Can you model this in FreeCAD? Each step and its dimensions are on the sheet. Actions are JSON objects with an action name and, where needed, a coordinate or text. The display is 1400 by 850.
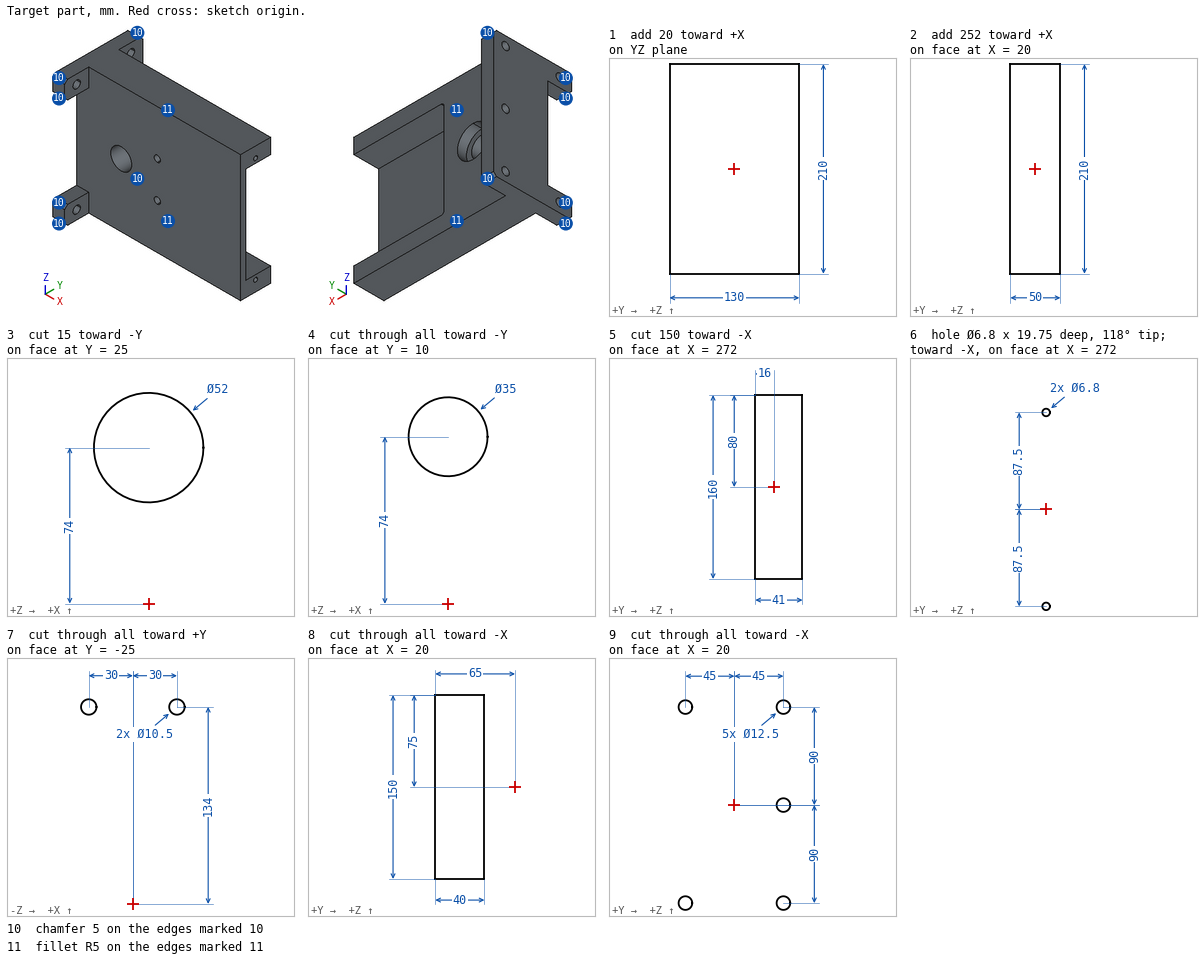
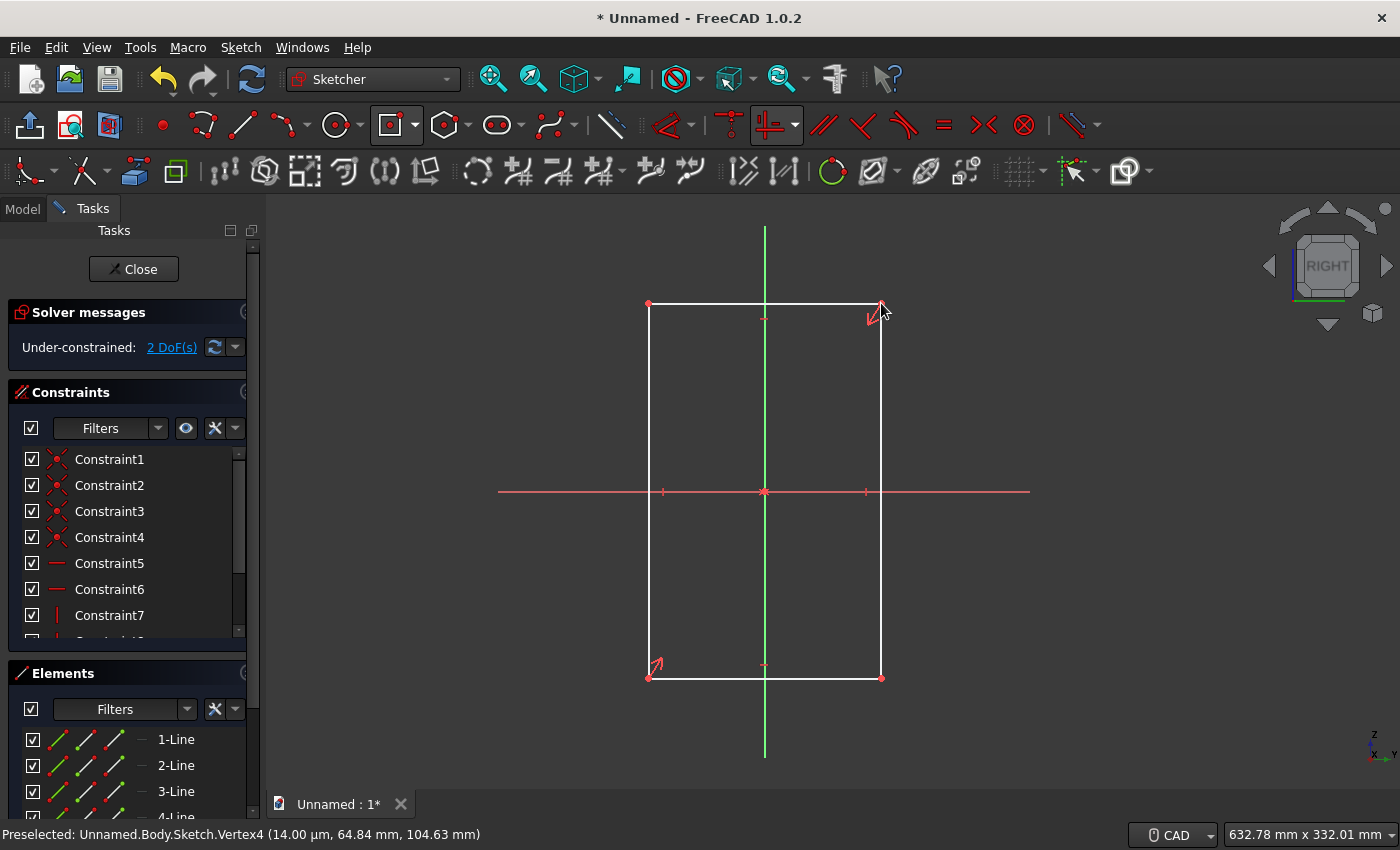
{"action": "left_click", "coordinate": [666, 126]}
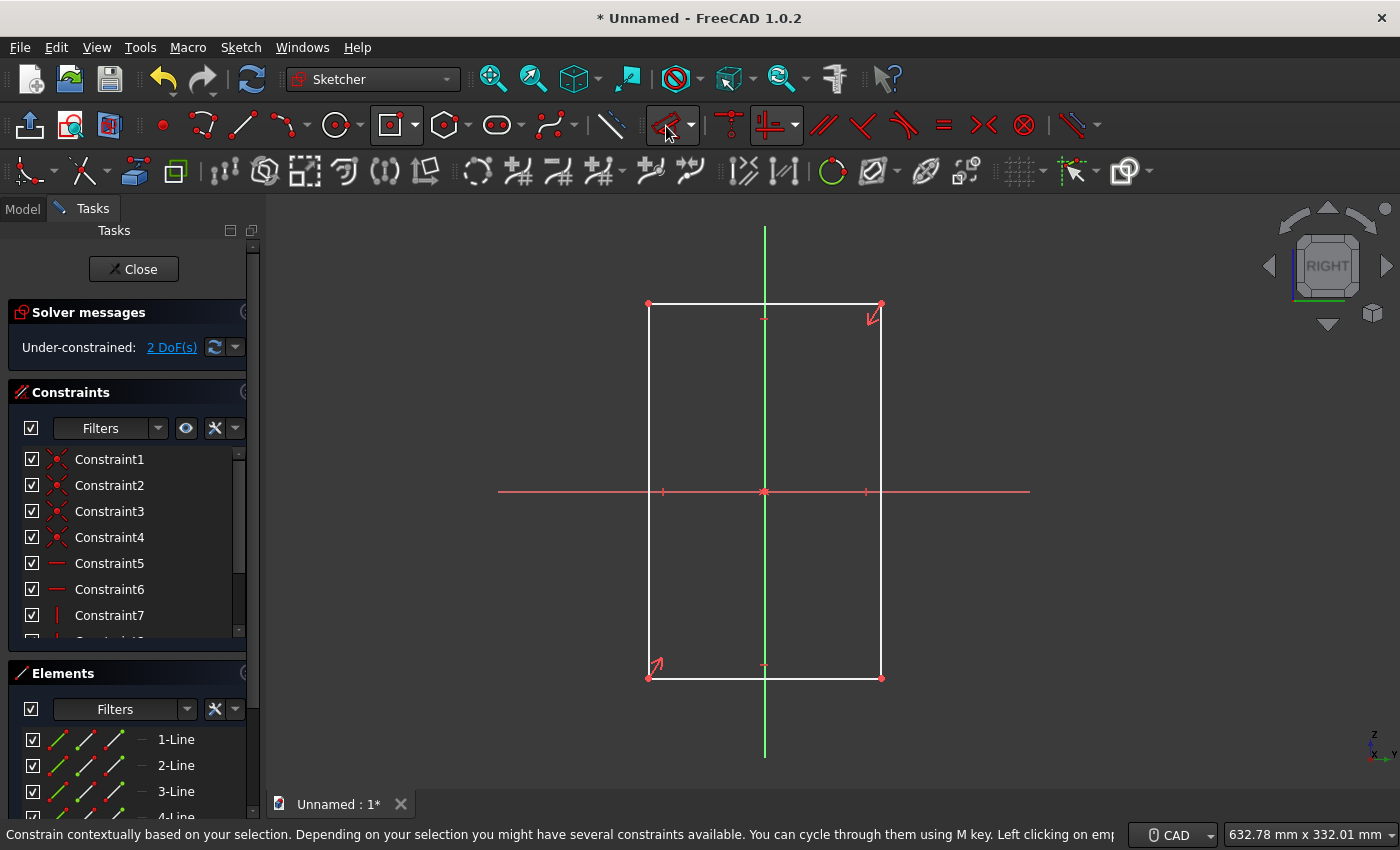
{"action": "left_click", "coordinate": [718, 679]}
{"action": "left_click", "coordinate": [711, 713]}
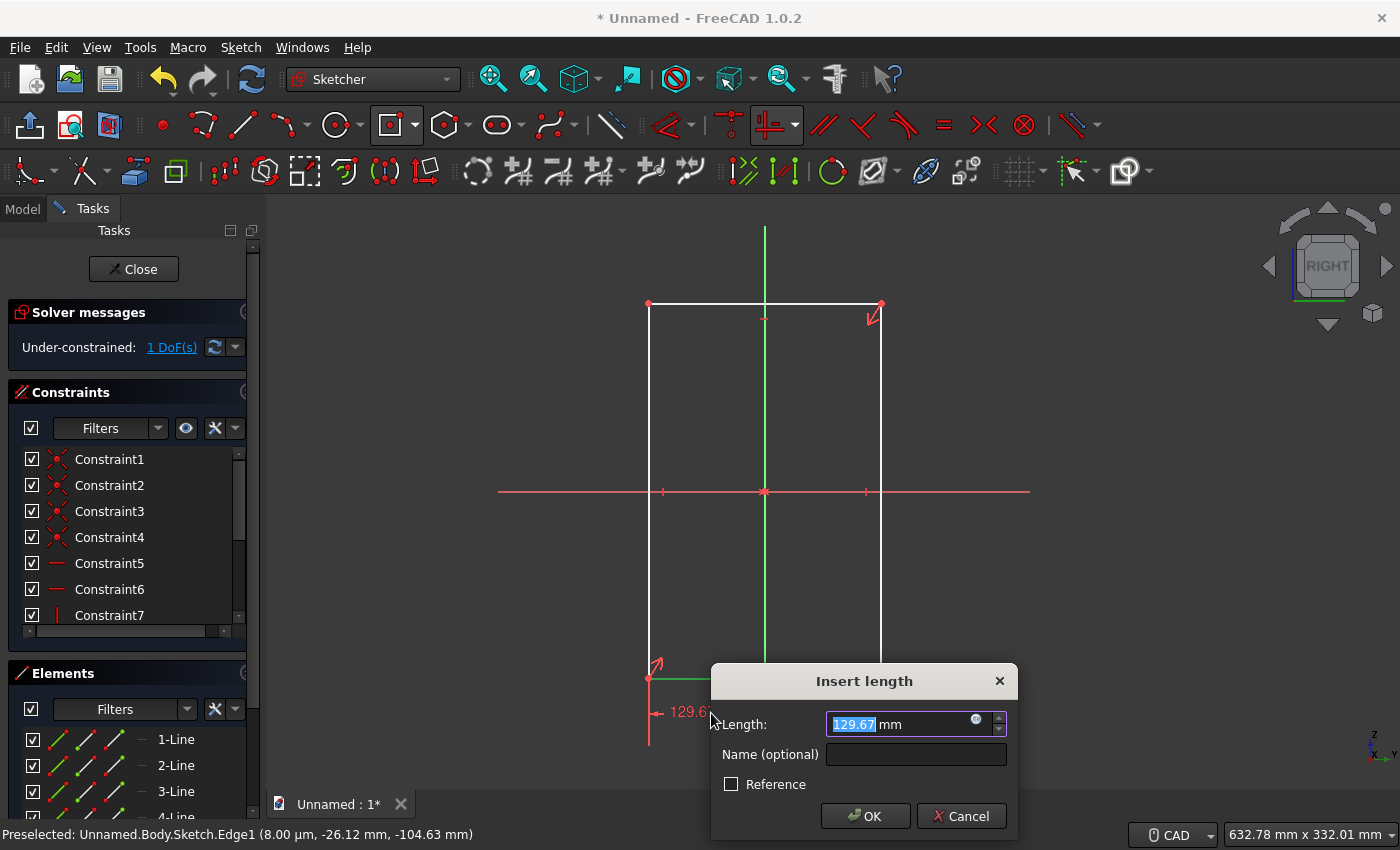
{"action": "type", "text": "130"}
{"action": "key", "text": "Return"}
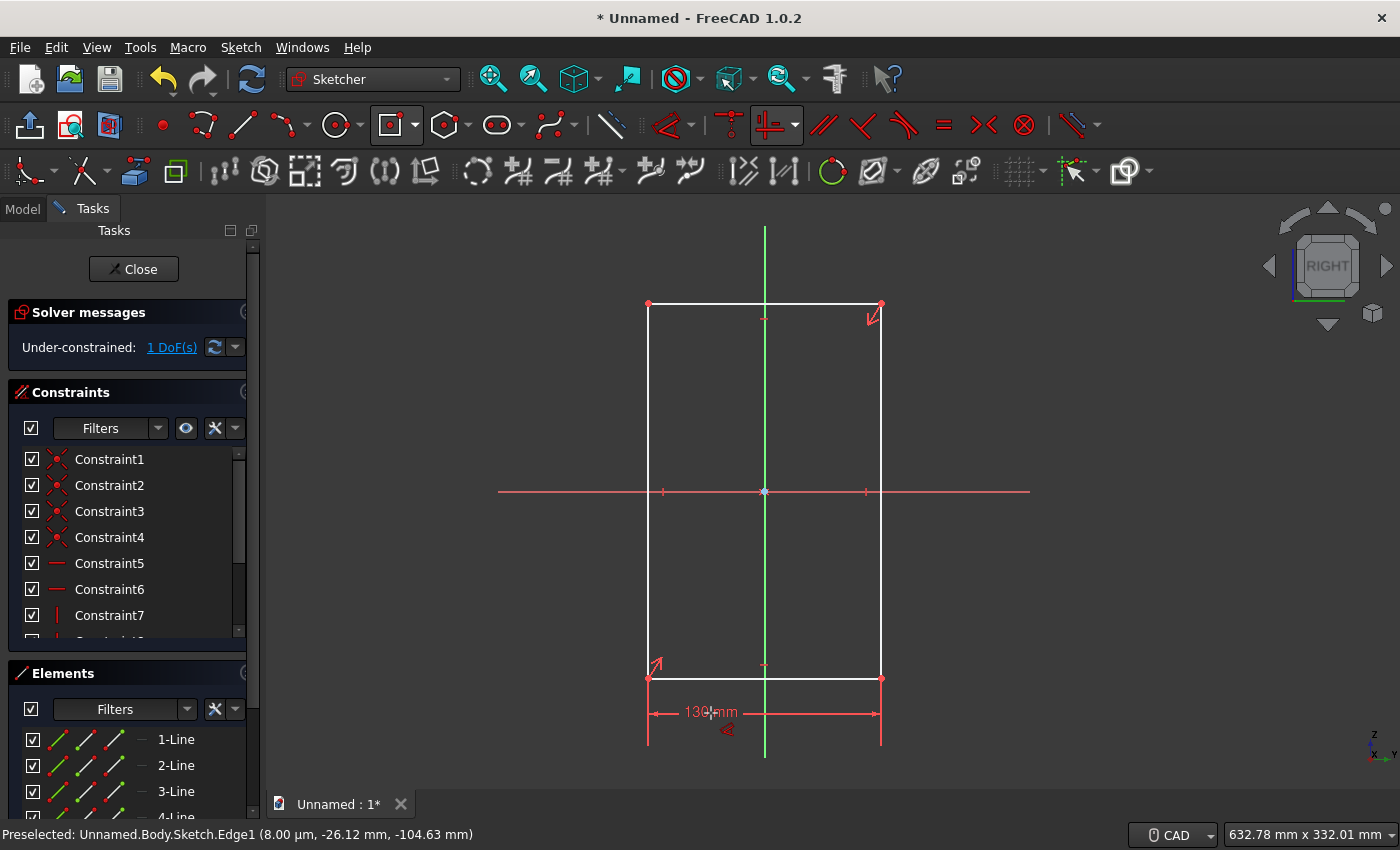
{"action": "left_click", "coordinate": [881, 567]}
{"action": "left_click", "coordinate": [915, 405]}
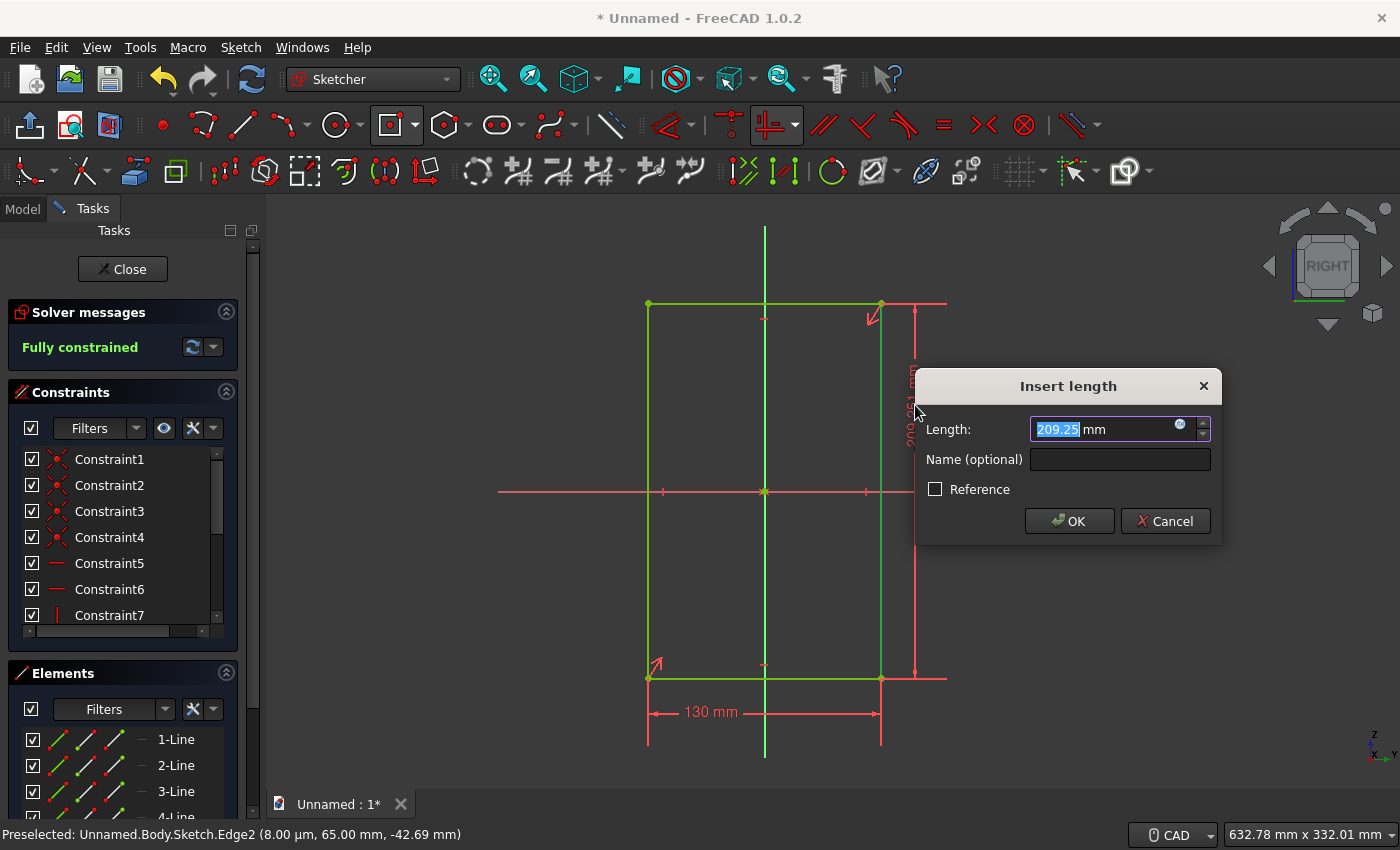
{"action": "type", "text": "210"}
{"action": "key", "text": "Return"}
{"action": "key", "text": "Escape"}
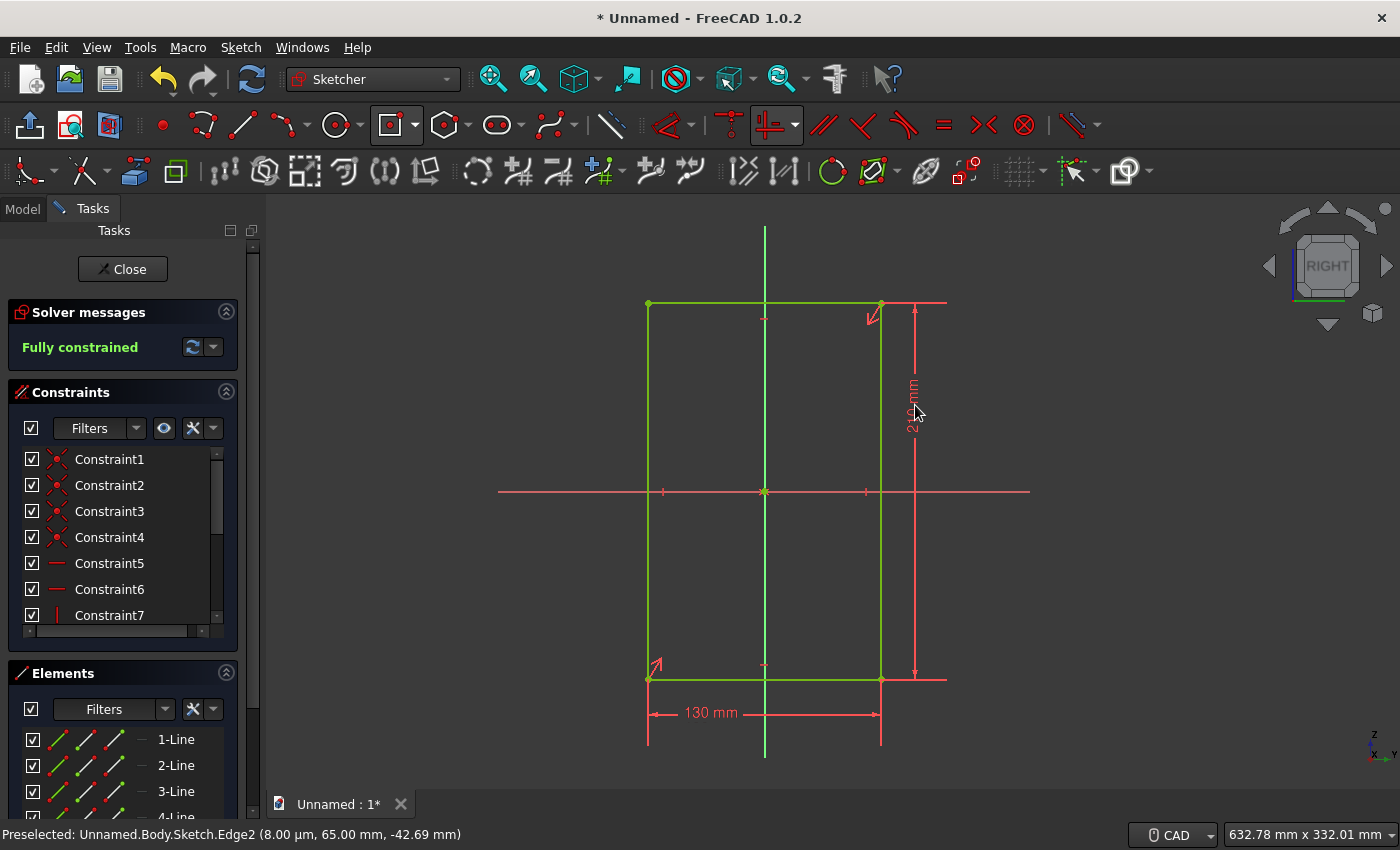
{"action": "left_click", "coordinate": [123, 269]}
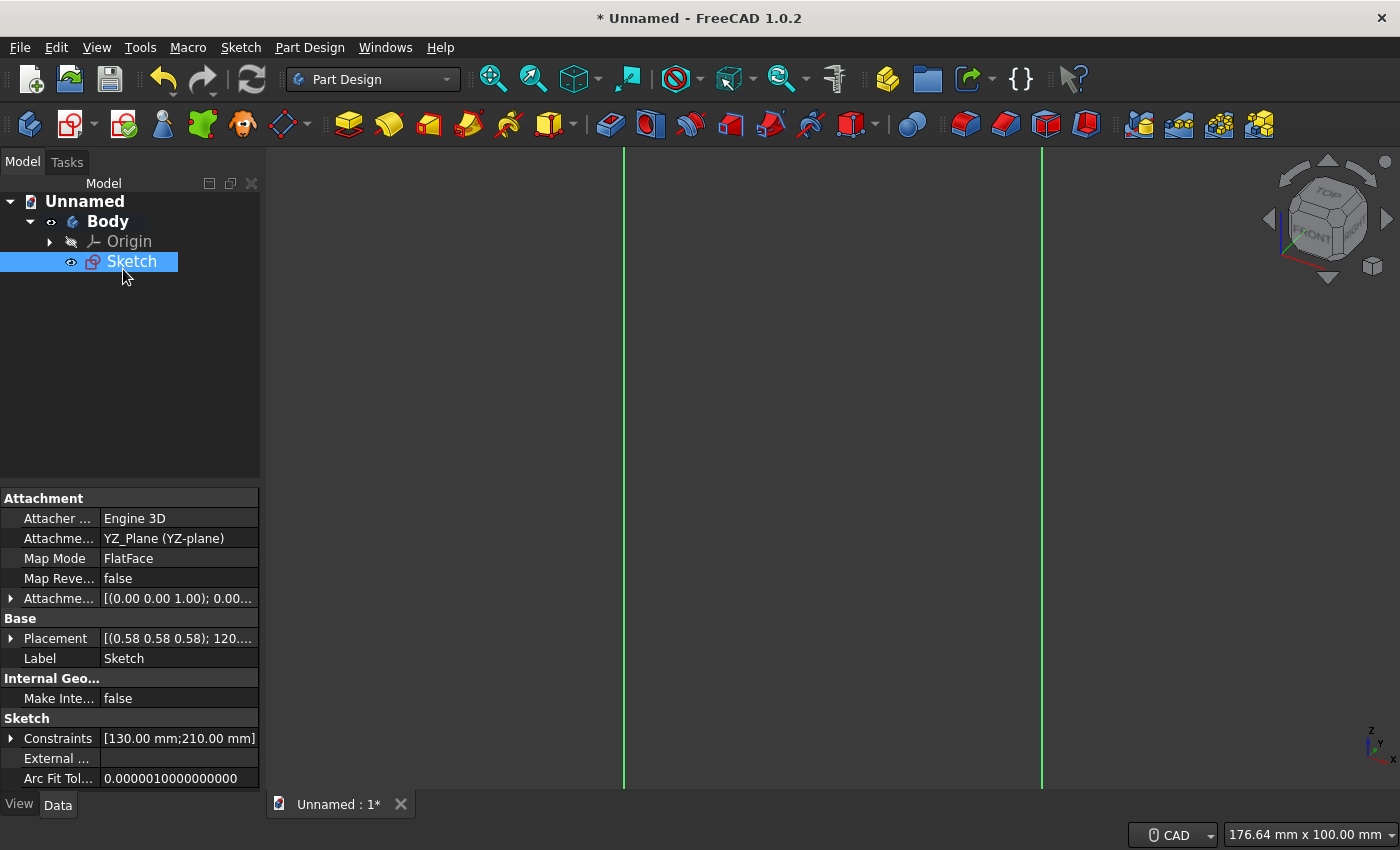
{"action": "left_click", "coordinate": [350, 124]}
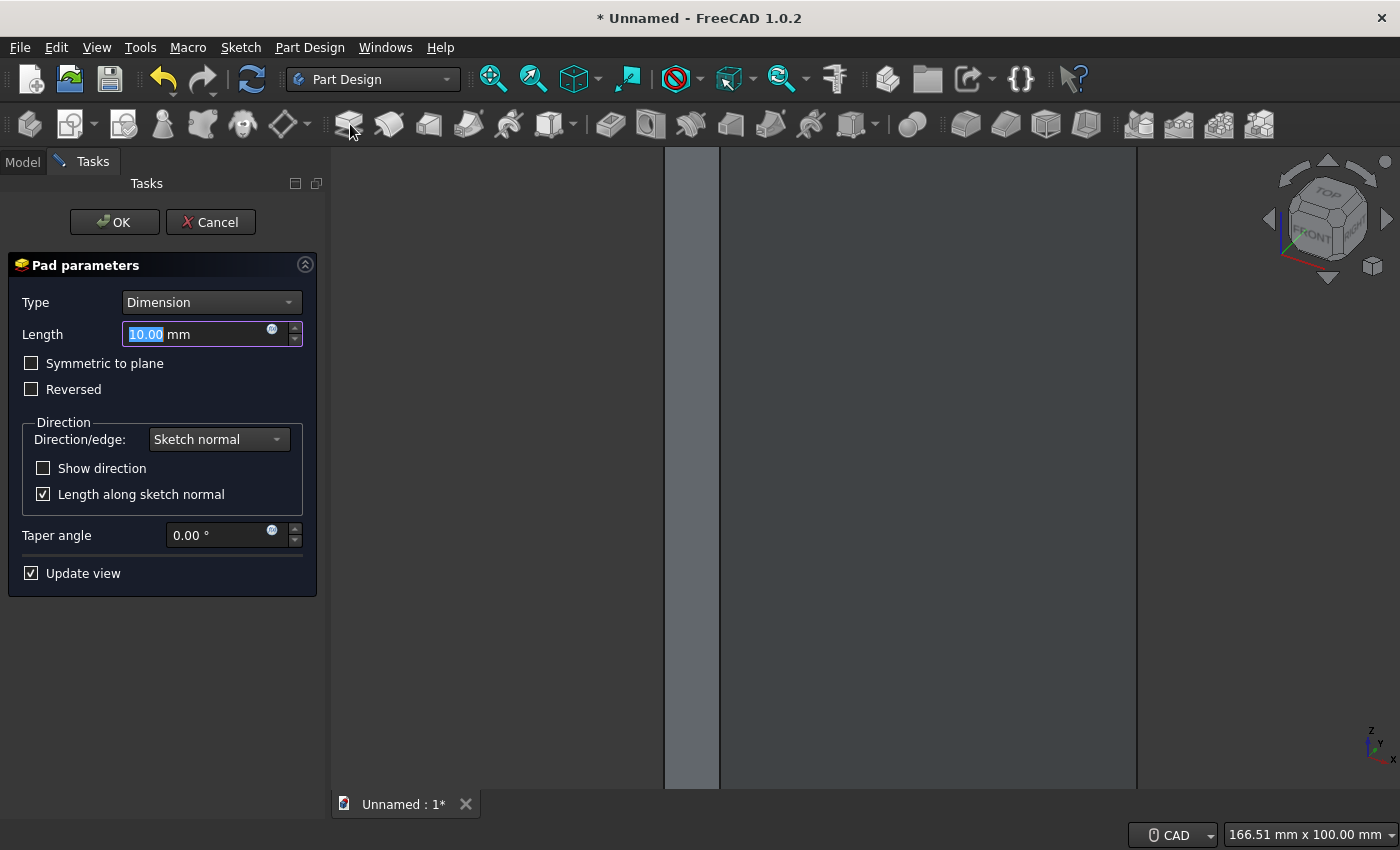
{"action": "type", "text": "20"}
{"action": "key", "text": "Tab"}